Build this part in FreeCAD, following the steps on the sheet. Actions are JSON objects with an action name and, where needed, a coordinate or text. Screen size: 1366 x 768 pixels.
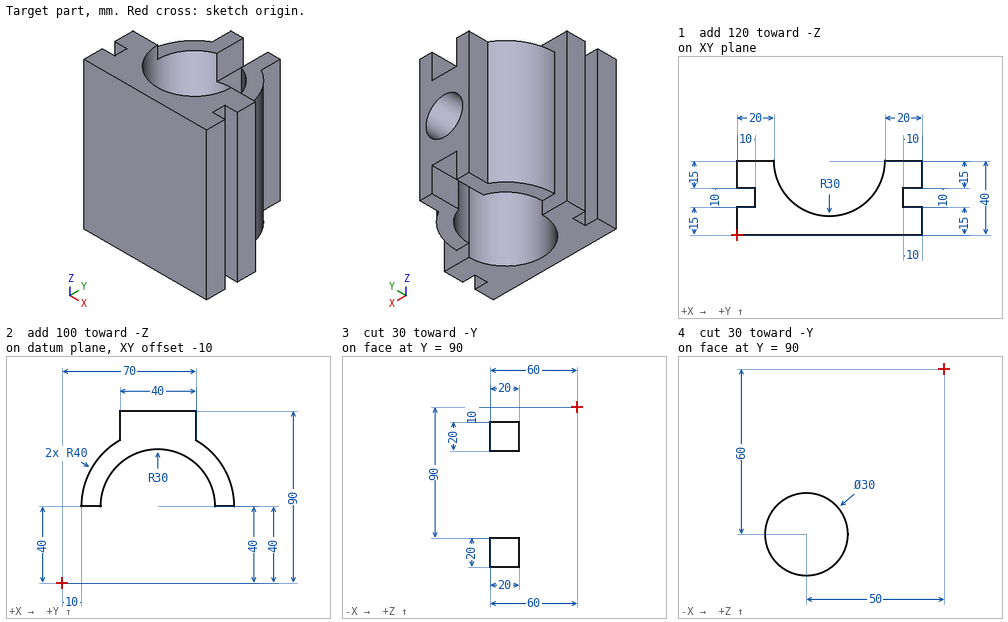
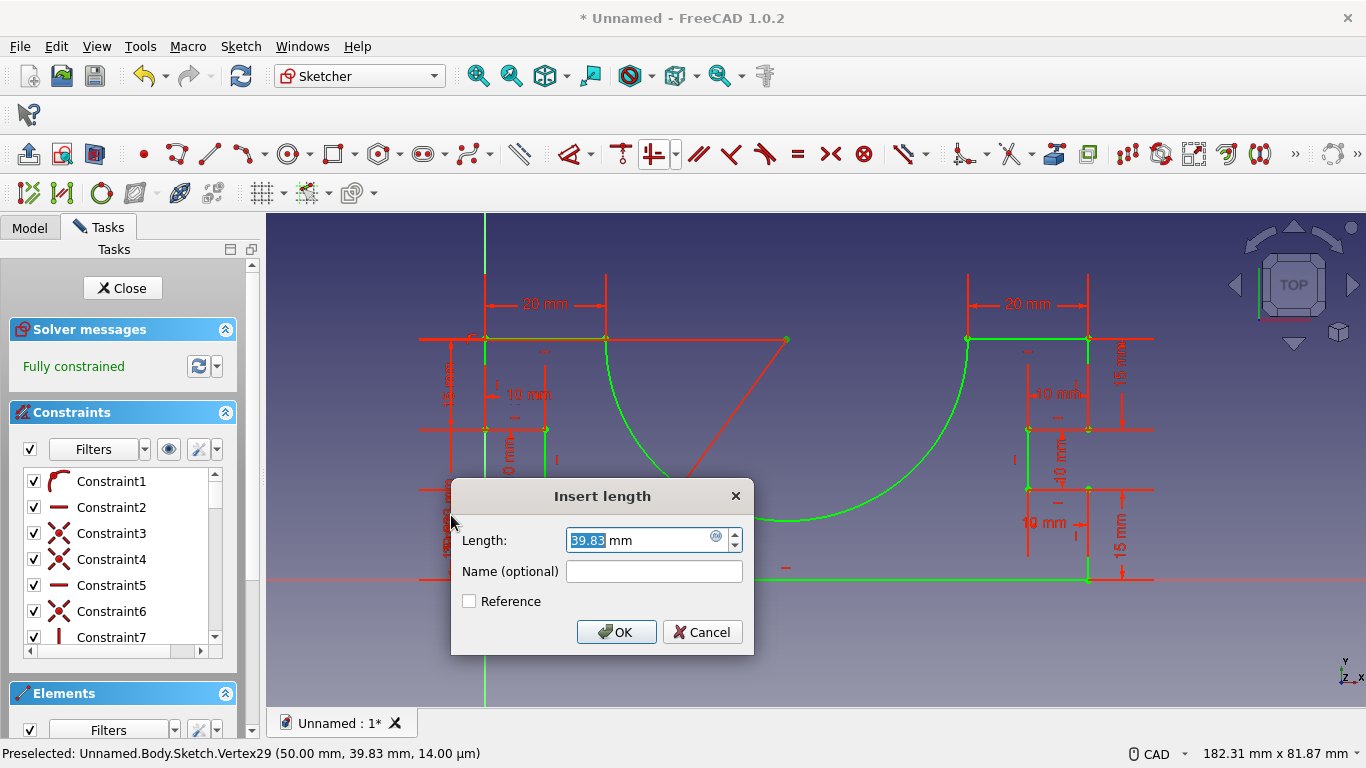
{"action": "type", "text": "40"}
{"action": "key", "text": "Return"}
{"action": "key", "text": "Escape"}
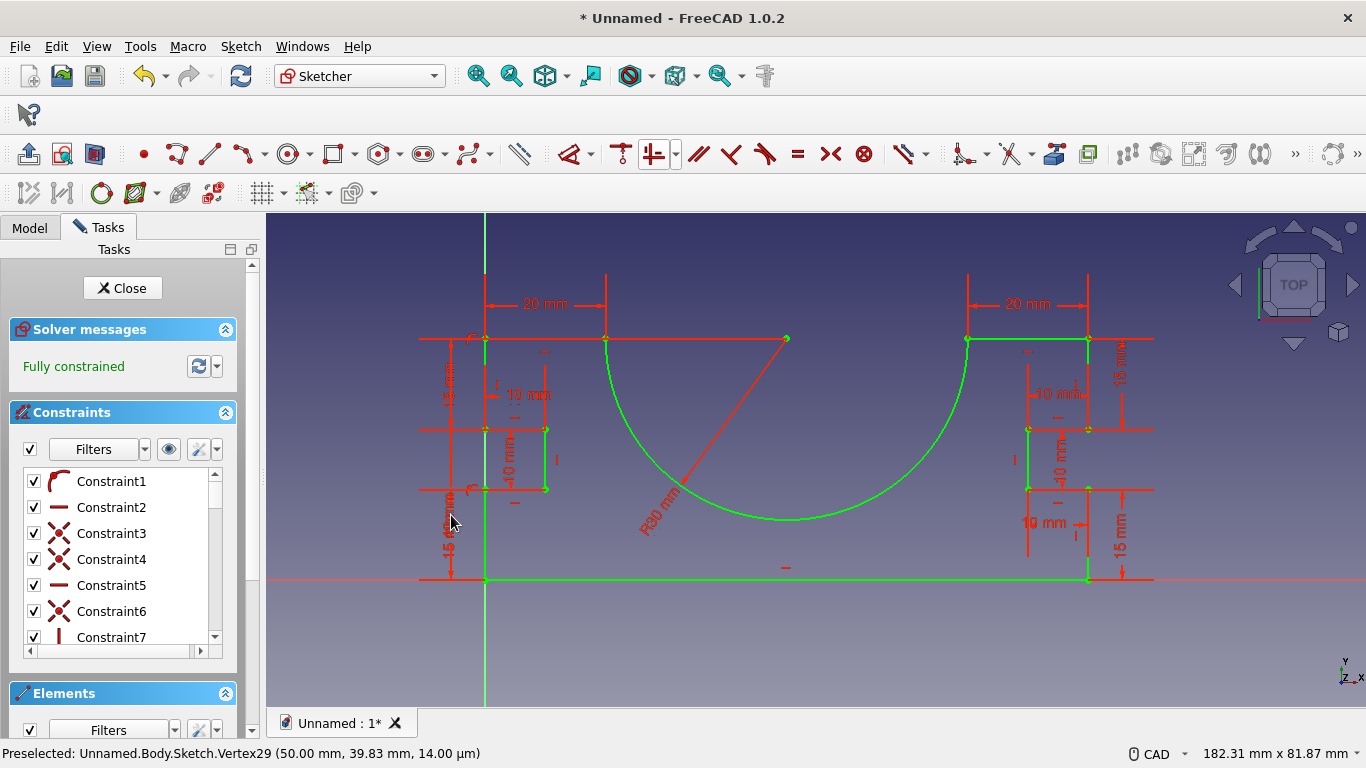
{"action": "left_click", "coordinate": [123, 288]}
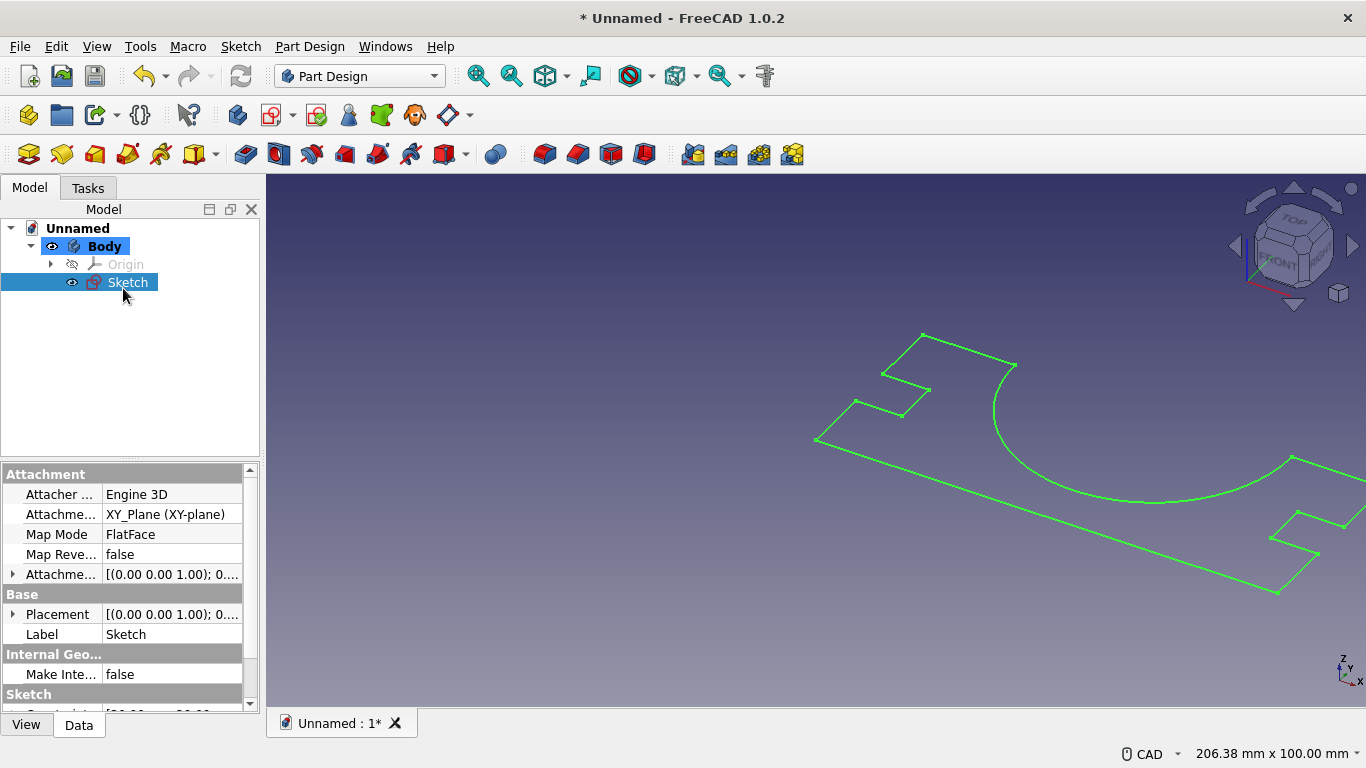
{"action": "left_click", "coordinate": [29, 154]}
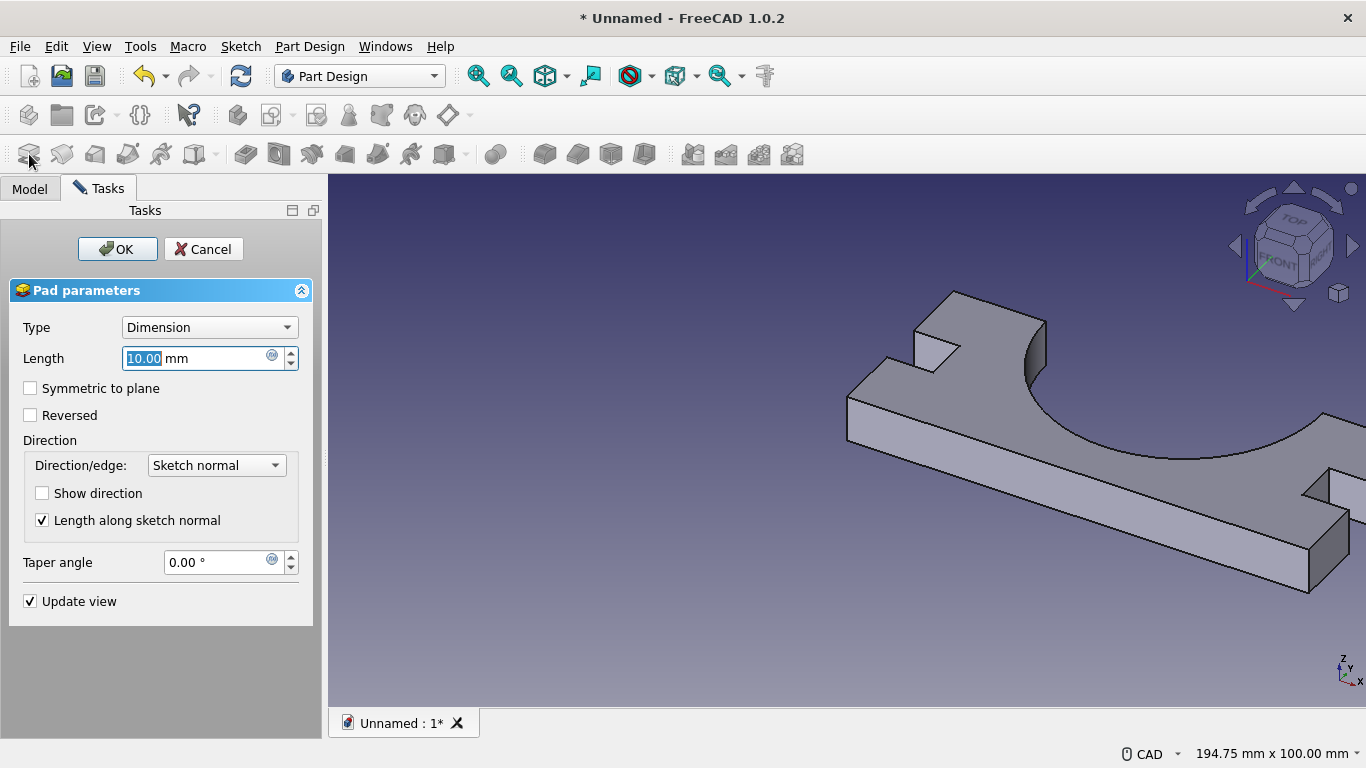
{"action": "type", "text": "120"}
{"action": "key", "text": "Tab"}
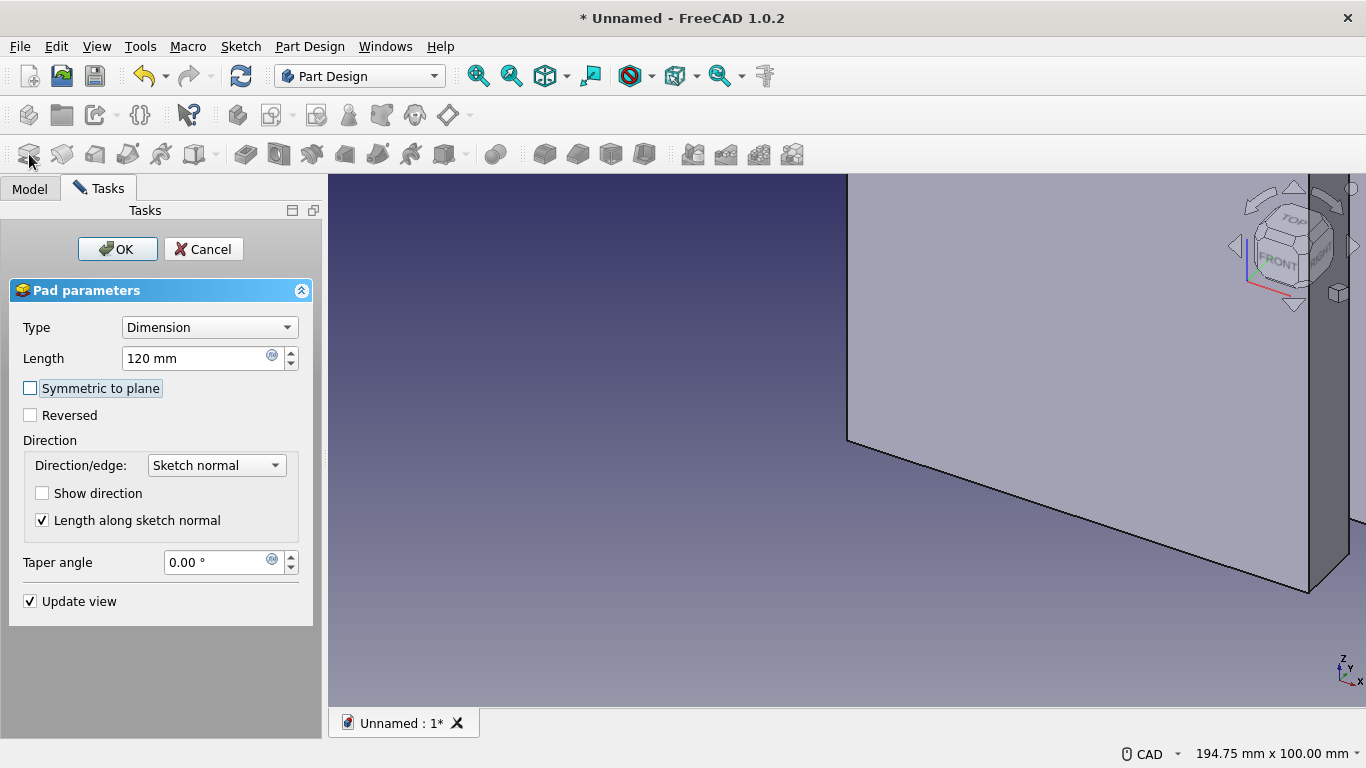
{"action": "left_click", "coordinate": [31, 415]}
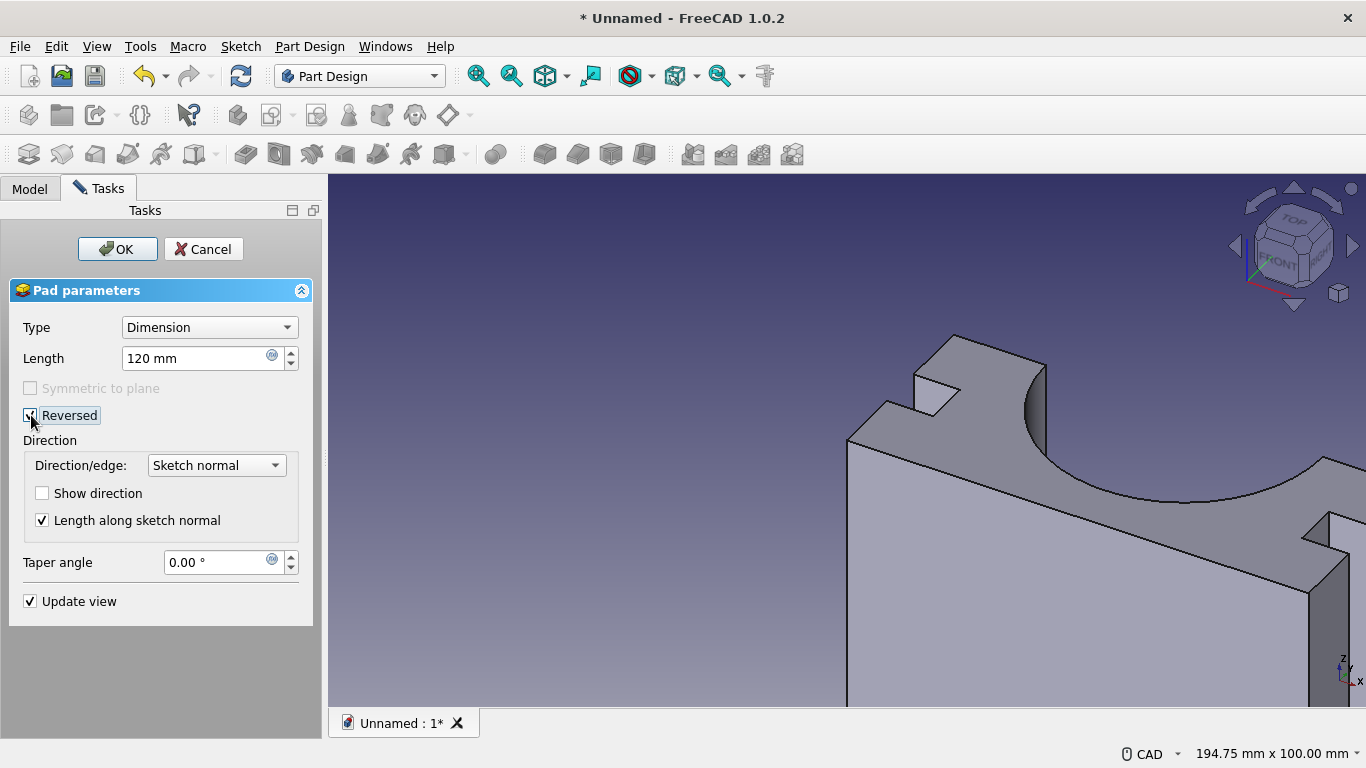
{"action": "left_click", "coordinate": [118, 249]}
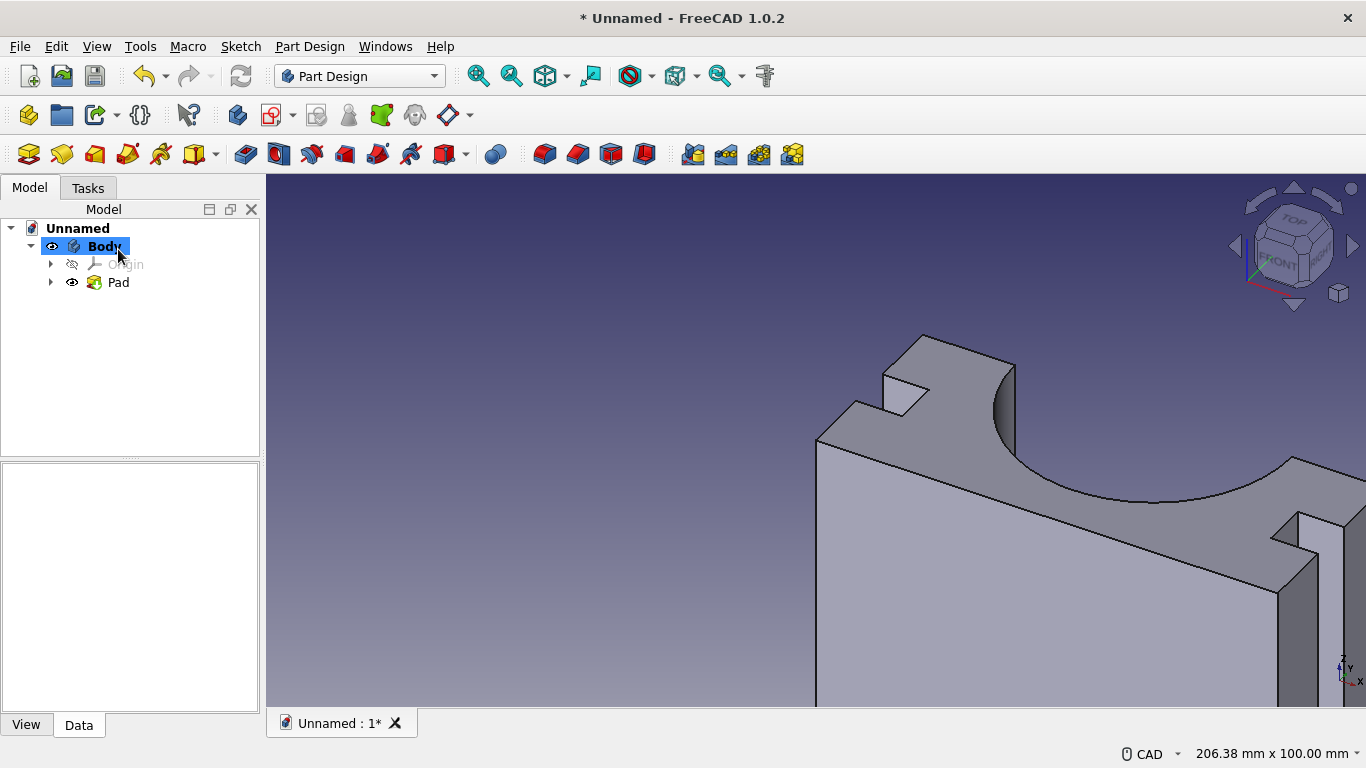
{"action": "left_click", "coordinate": [479, 76]}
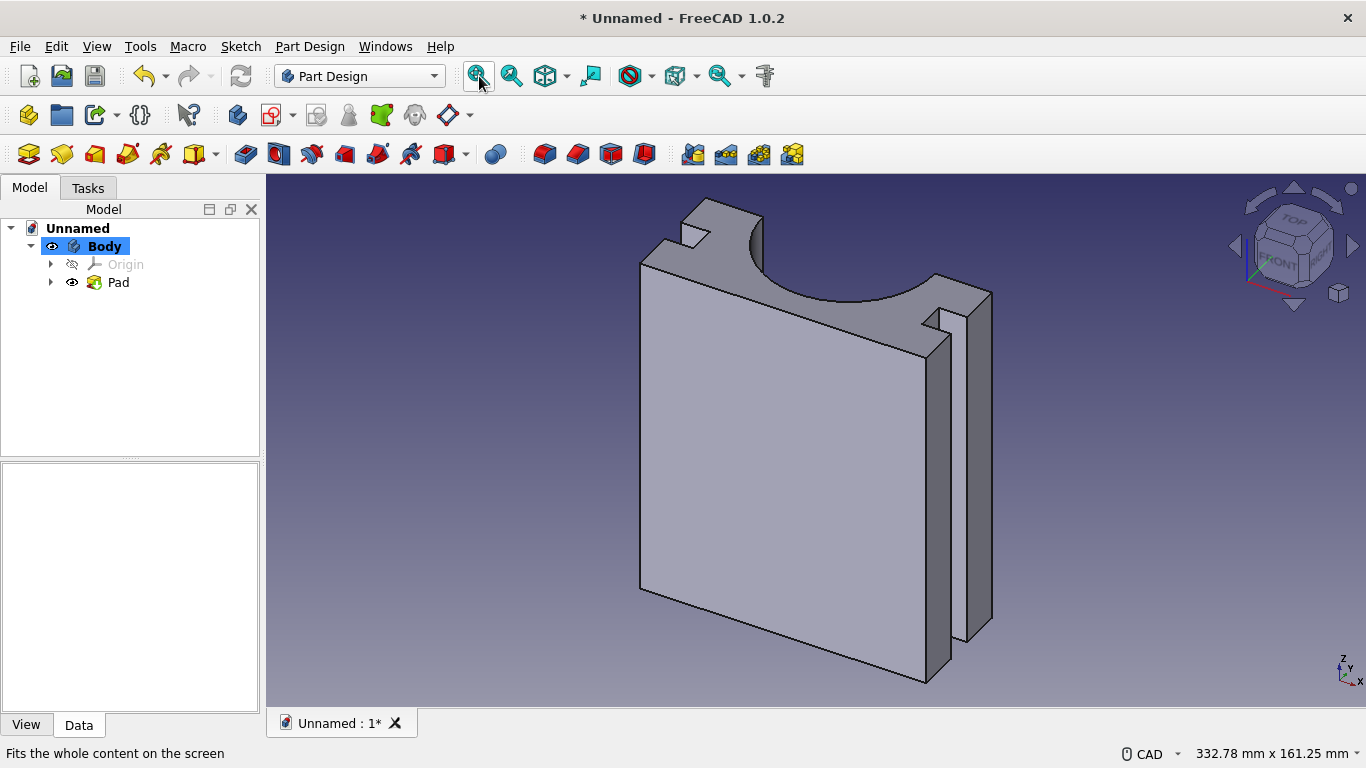
{"action": "left_click", "coordinate": [51, 264]}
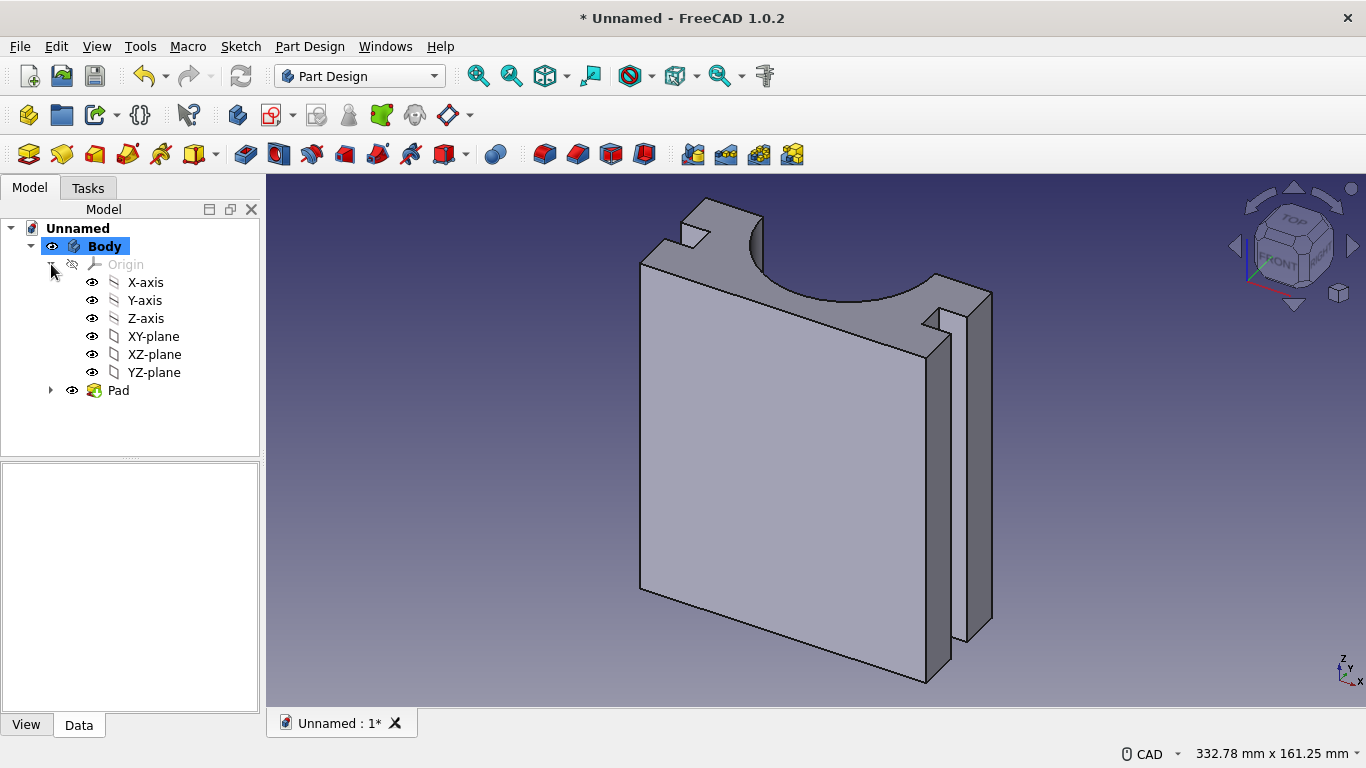
{"action": "left_click", "coordinate": [137, 336]}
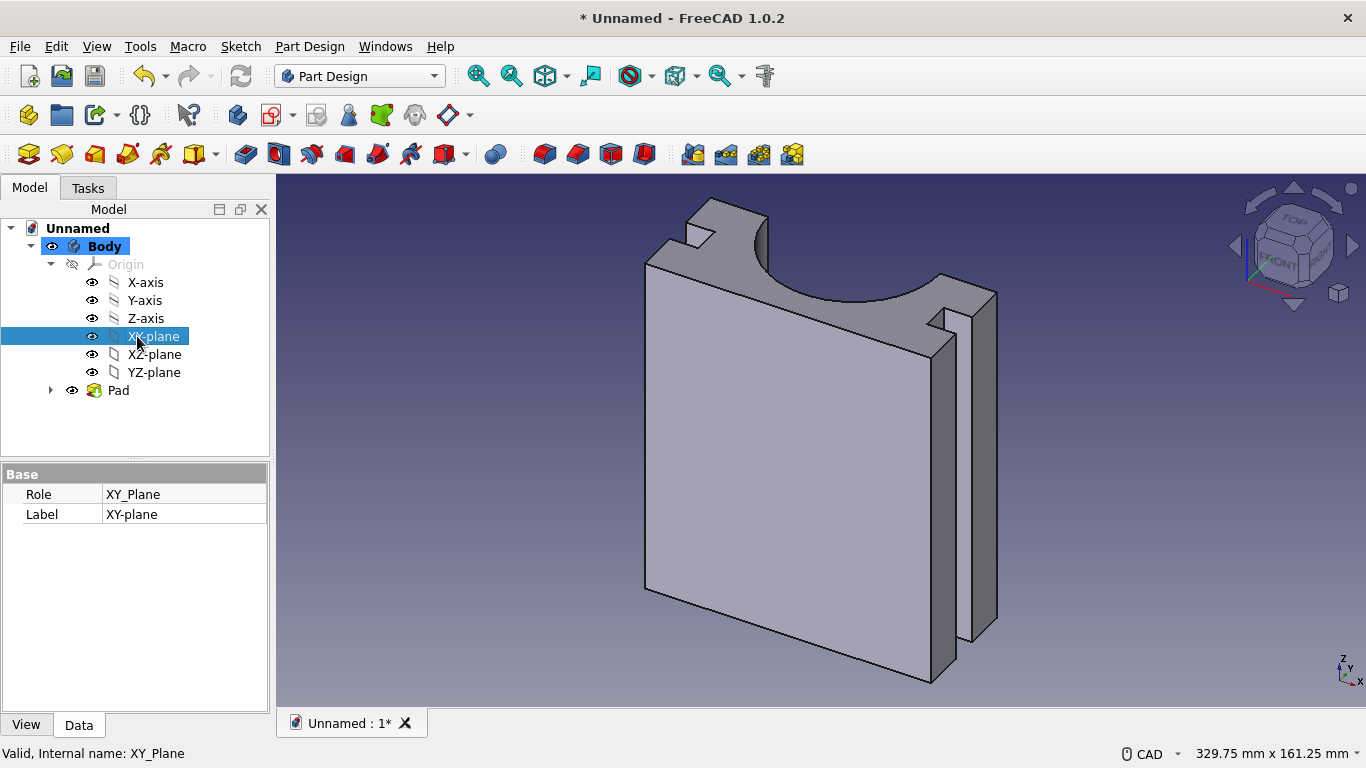
{"action": "left_click", "coordinate": [448, 116]}